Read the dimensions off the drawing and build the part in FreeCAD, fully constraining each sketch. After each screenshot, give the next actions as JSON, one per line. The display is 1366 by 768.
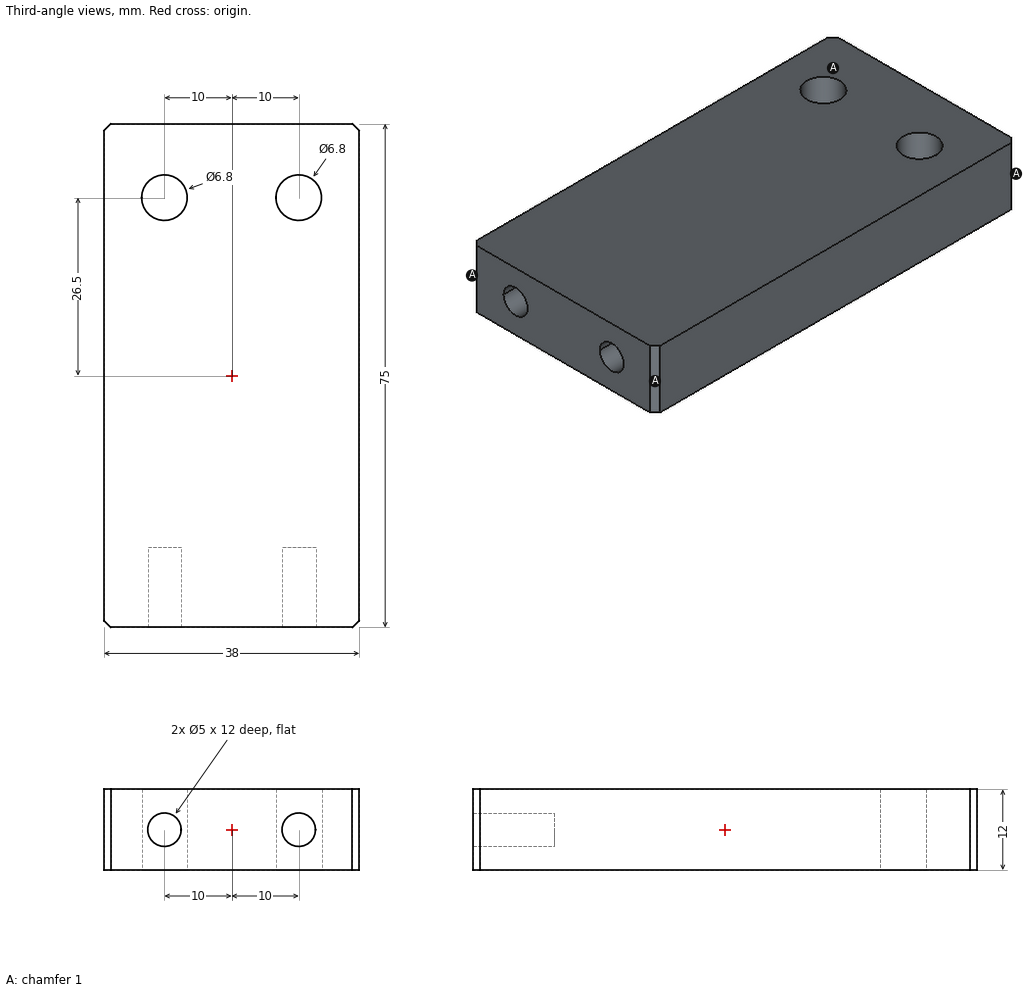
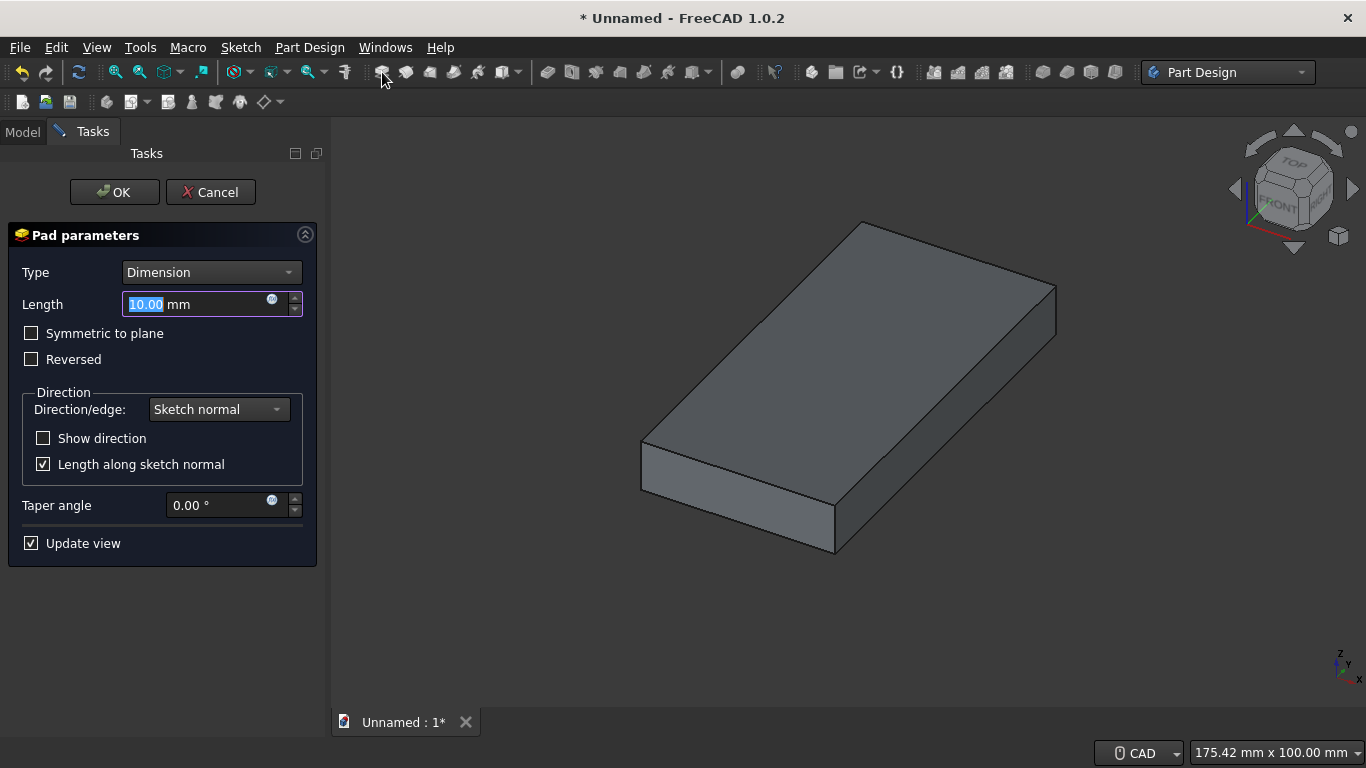
{"action": "type", "text": "12"}
{"action": "key", "text": "Tab"}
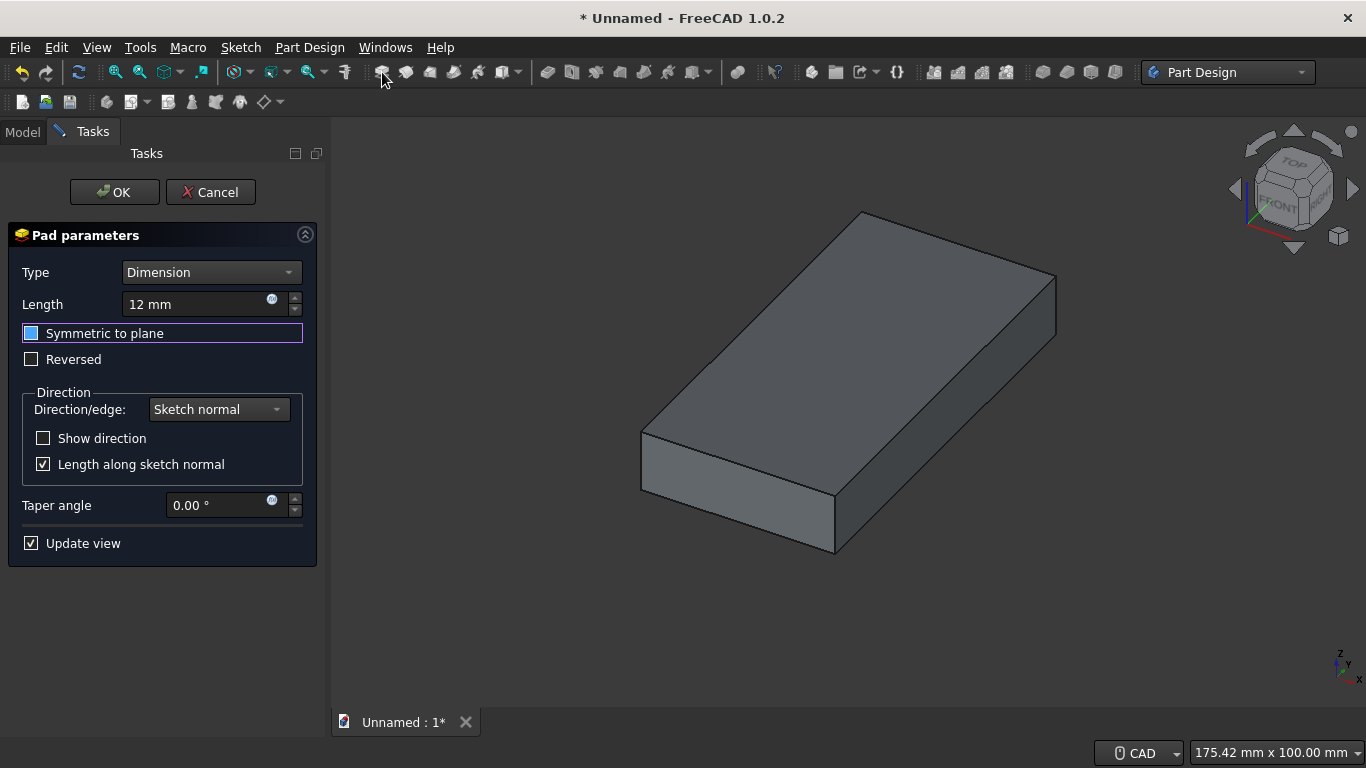
{"action": "left_click", "coordinate": [30, 333]}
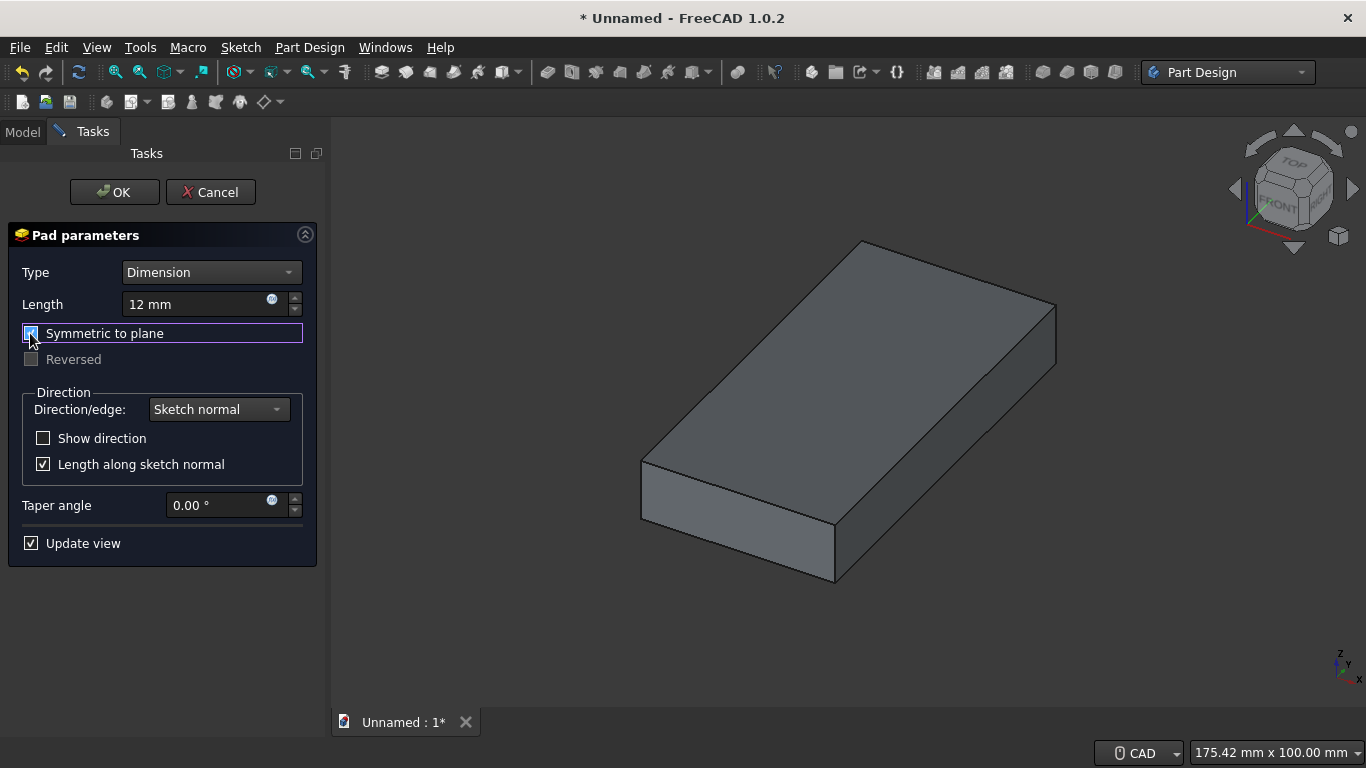
{"action": "left_click", "coordinate": [115, 192]}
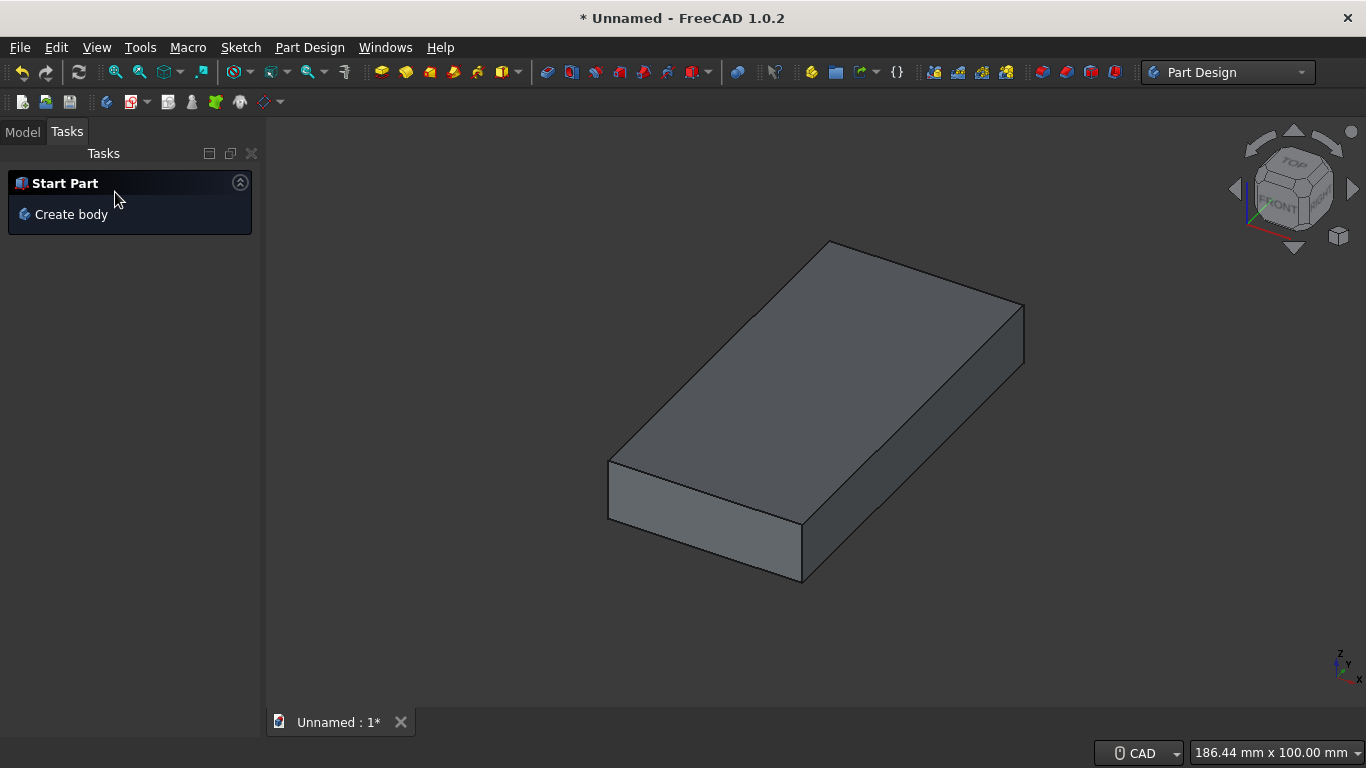
{"action": "left_click", "coordinate": [848, 351]}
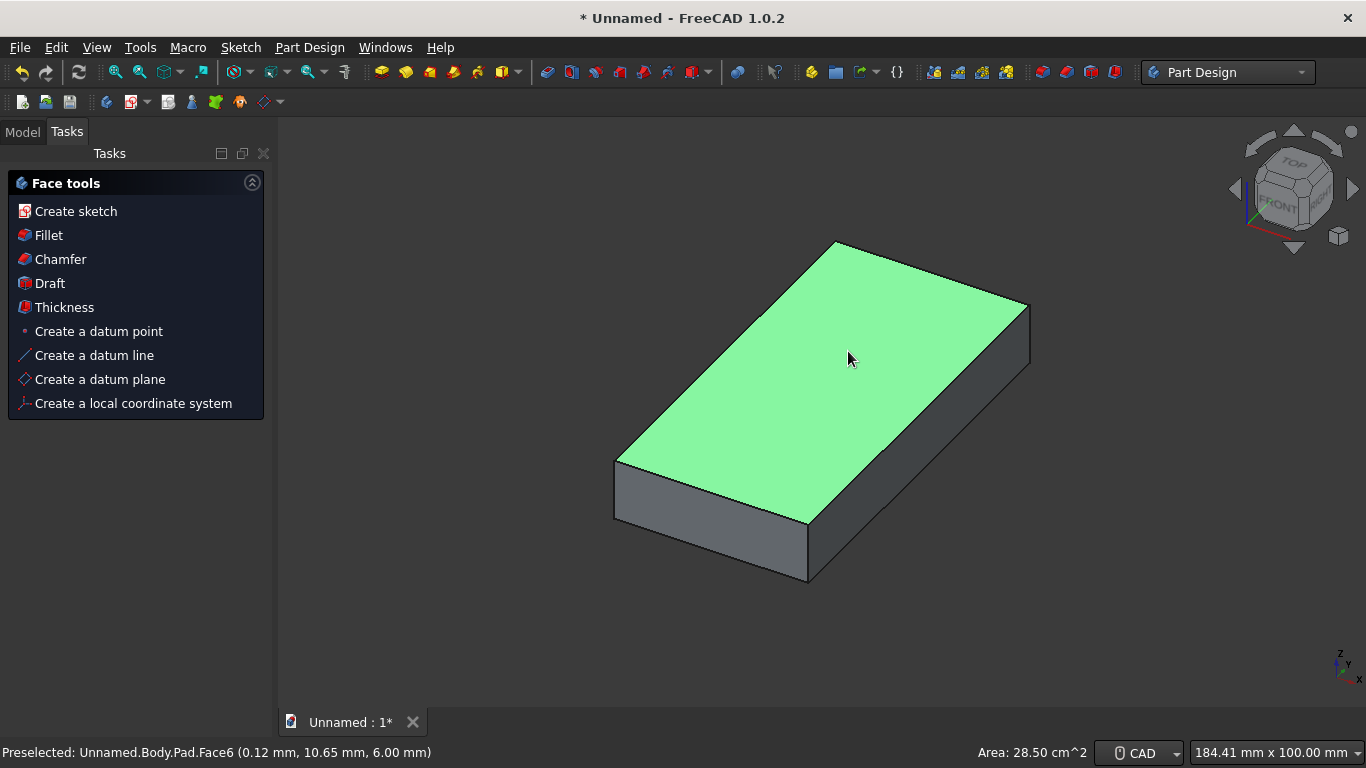
{"action": "left_click", "coordinate": [132, 102]}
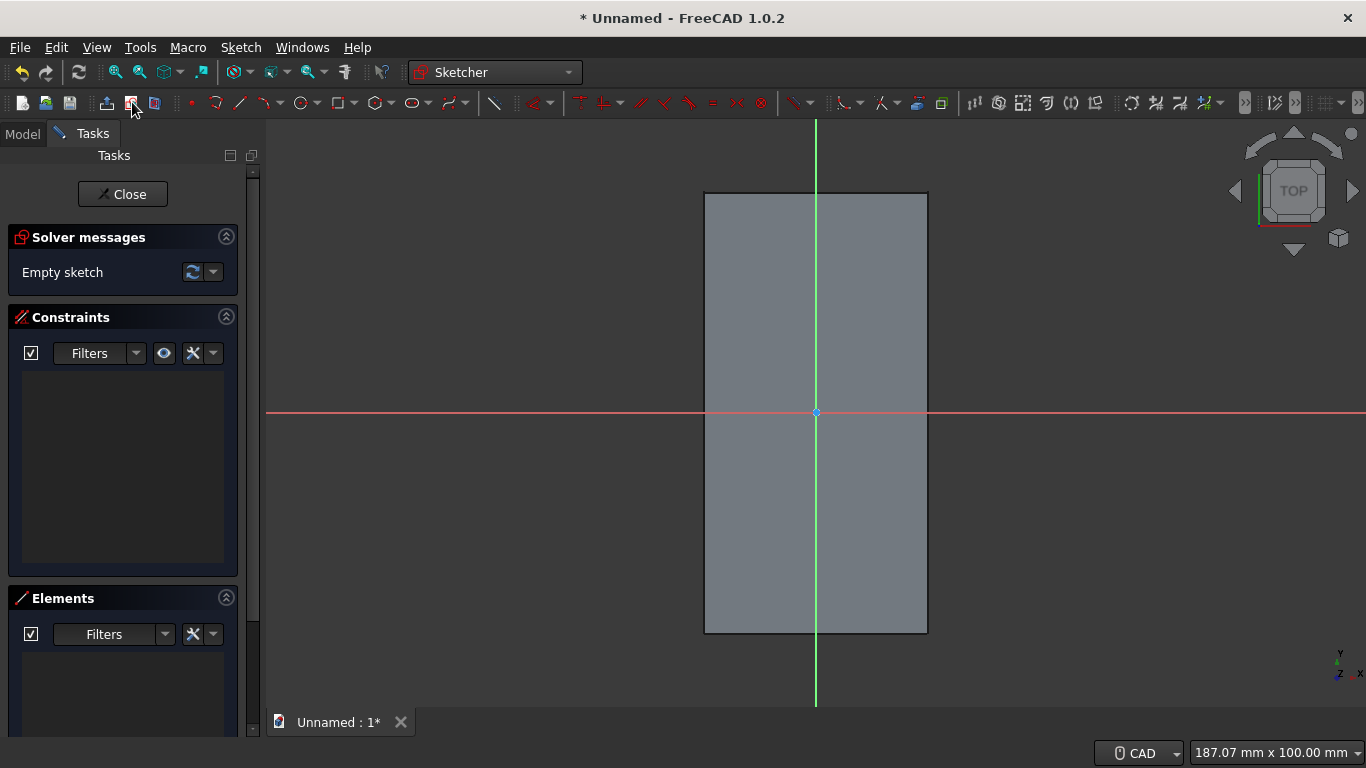
{"action": "scroll", "coordinate": [758, 238], "scroll_direction": "up", "scroll_amount": 11}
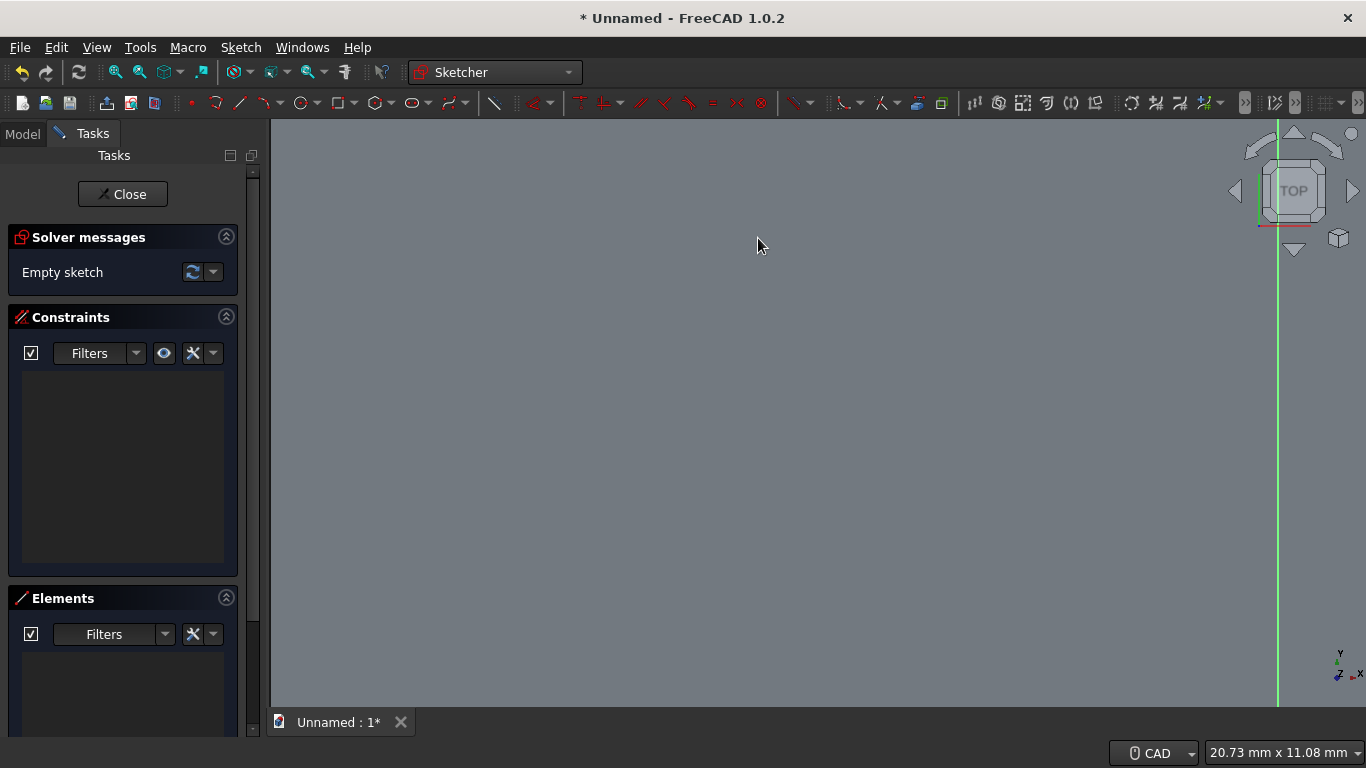
{"action": "key", "text": "g c"}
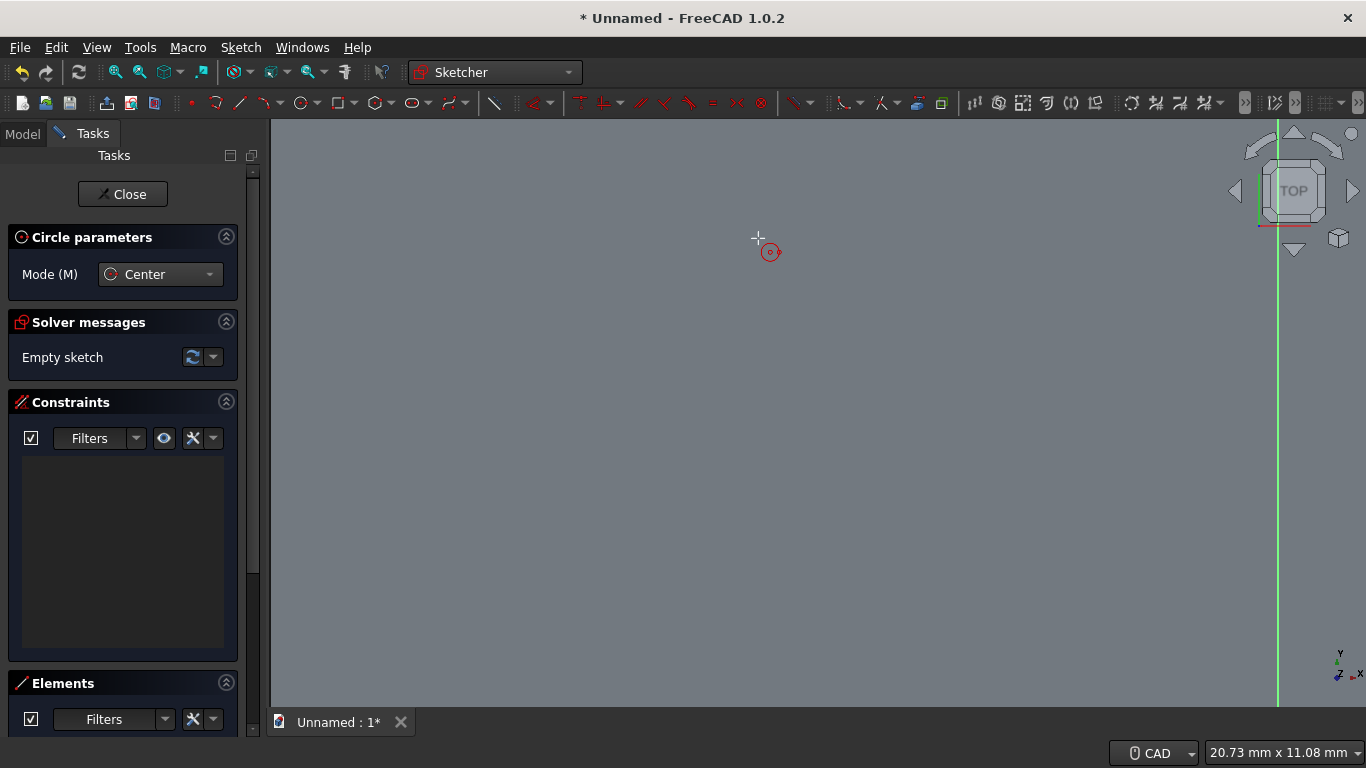
{"action": "left_click", "coordinate": [747, 409]}
{"action": "mouse_move", "coordinate": [875, 282]}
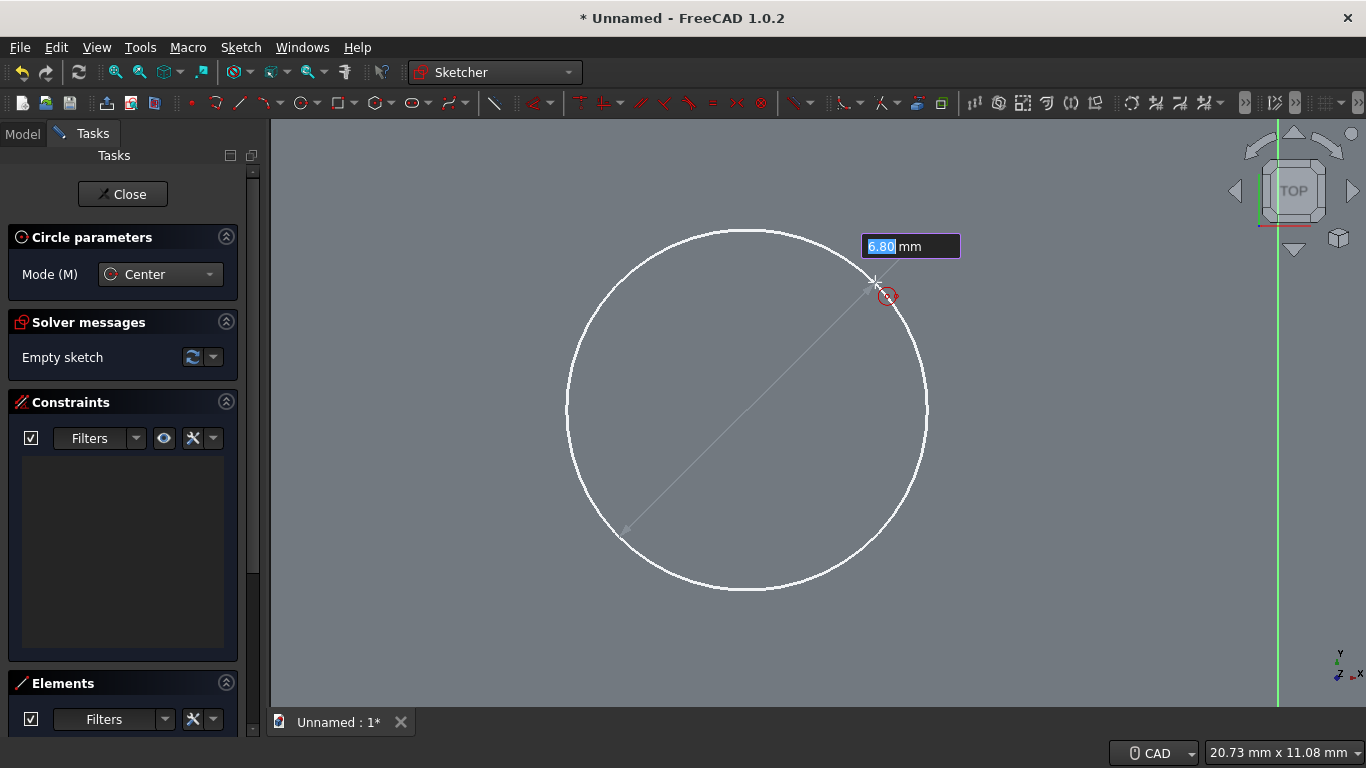
{"action": "type", "text": "6.8"}
{"action": "key", "text": "Return"}
{"action": "key", "text": "Escape"}